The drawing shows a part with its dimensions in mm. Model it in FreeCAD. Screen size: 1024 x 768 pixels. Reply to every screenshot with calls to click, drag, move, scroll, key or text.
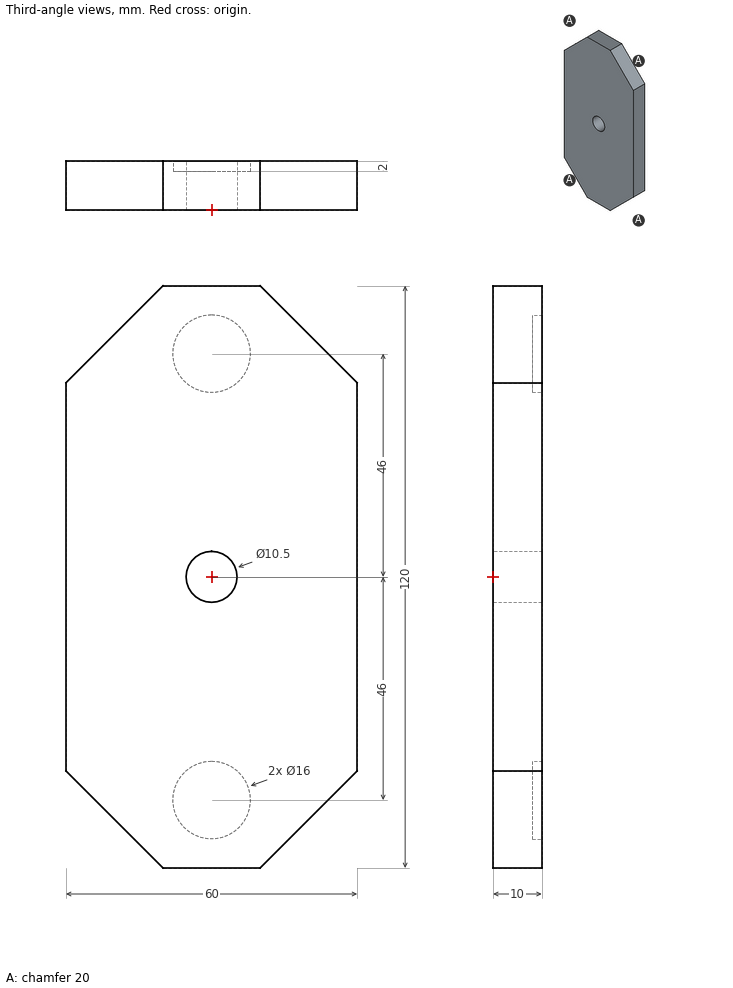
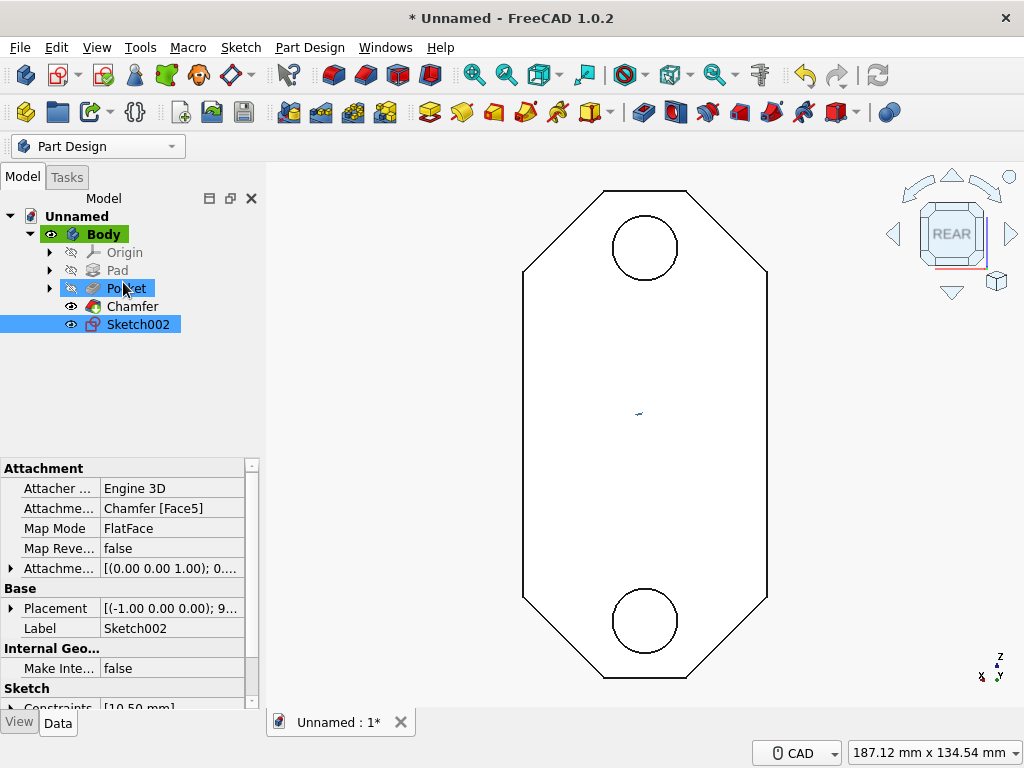
click(644, 112)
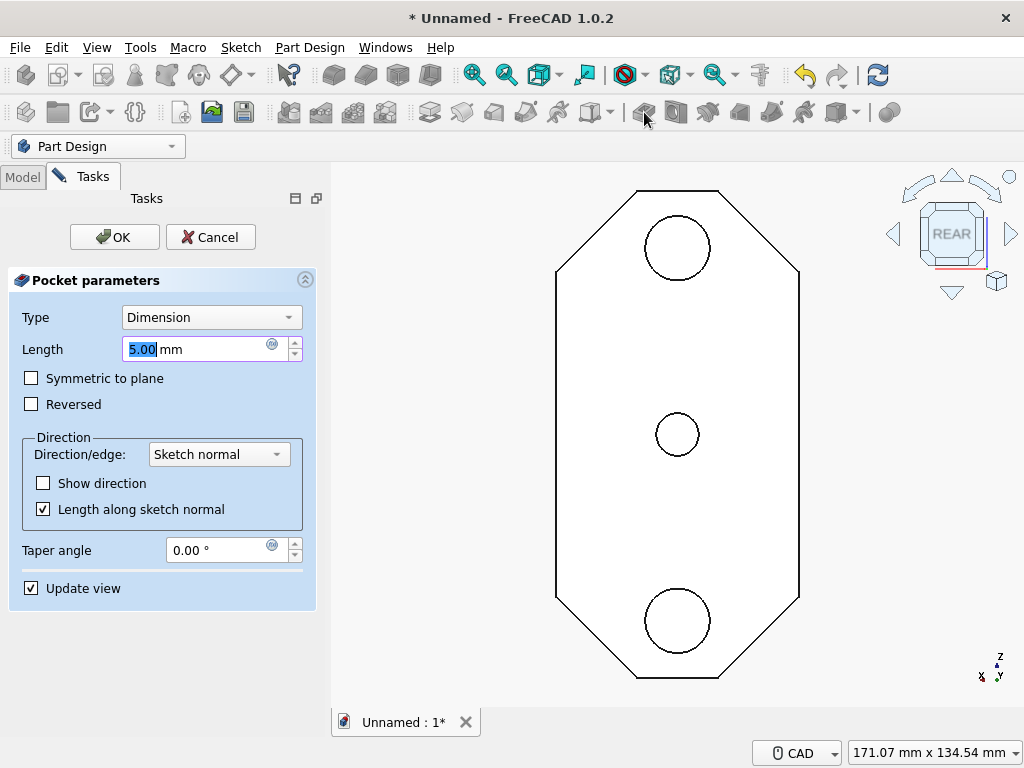
click(212, 318)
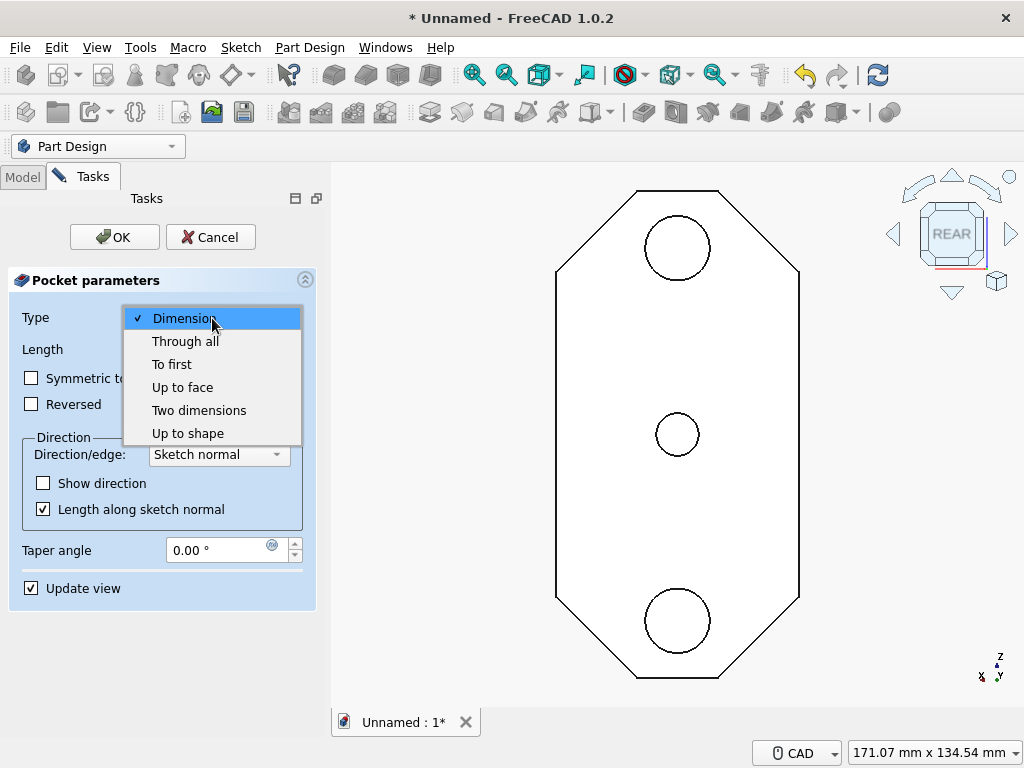
click(212, 364)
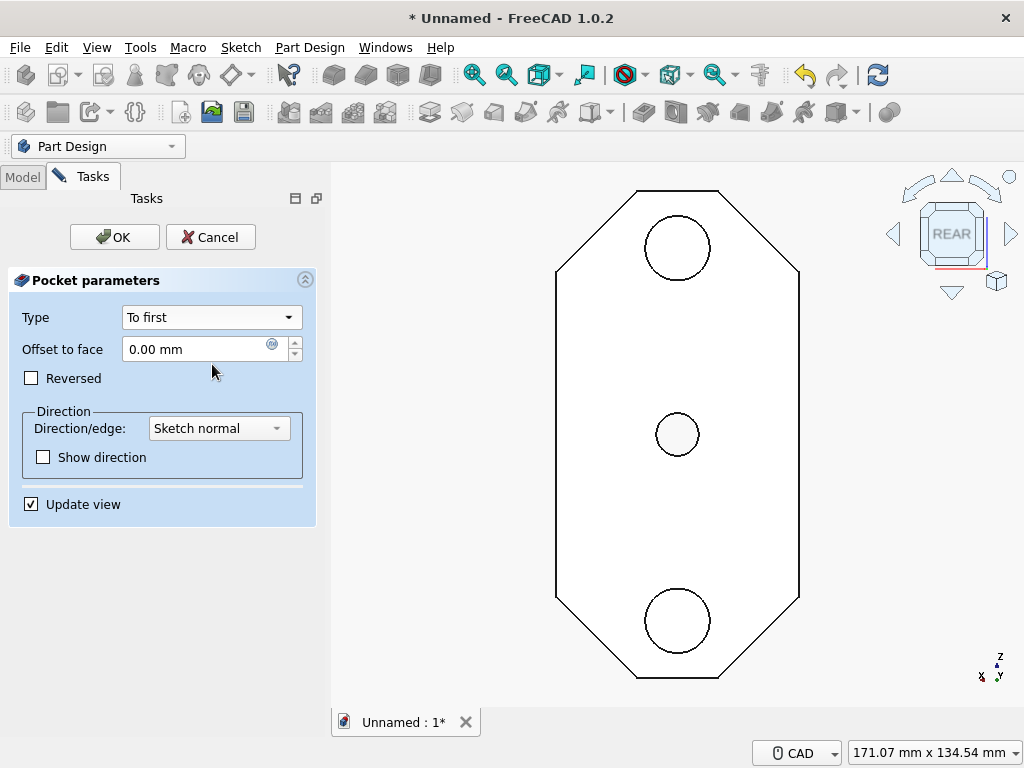
click(115, 237)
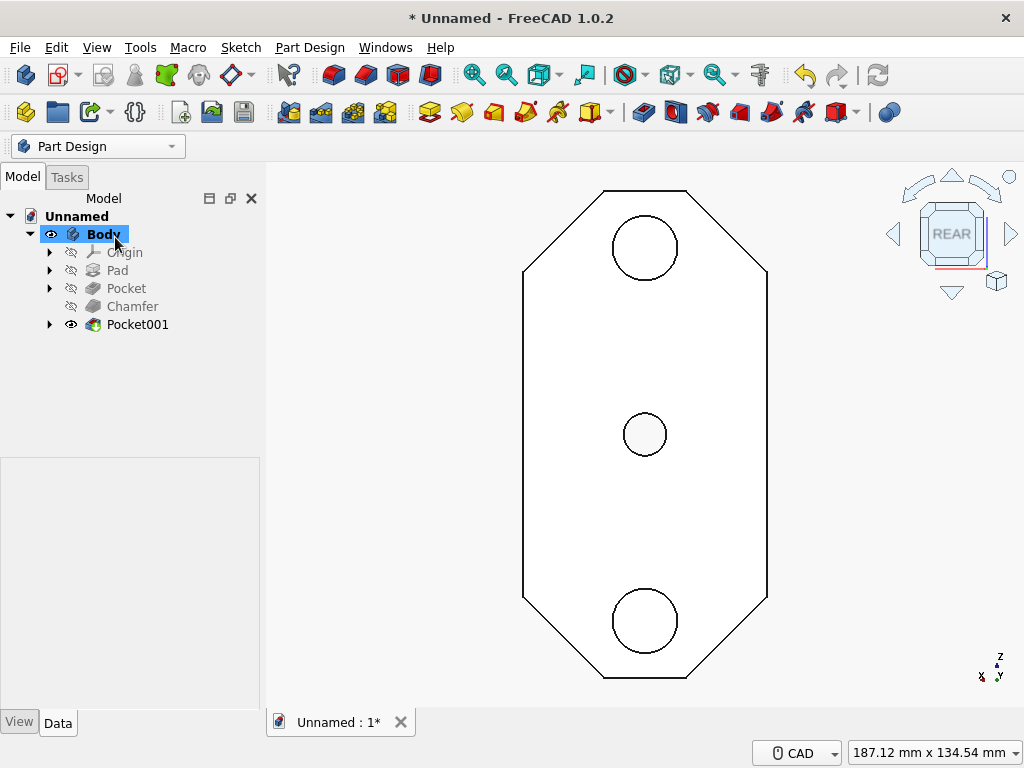
key(0)